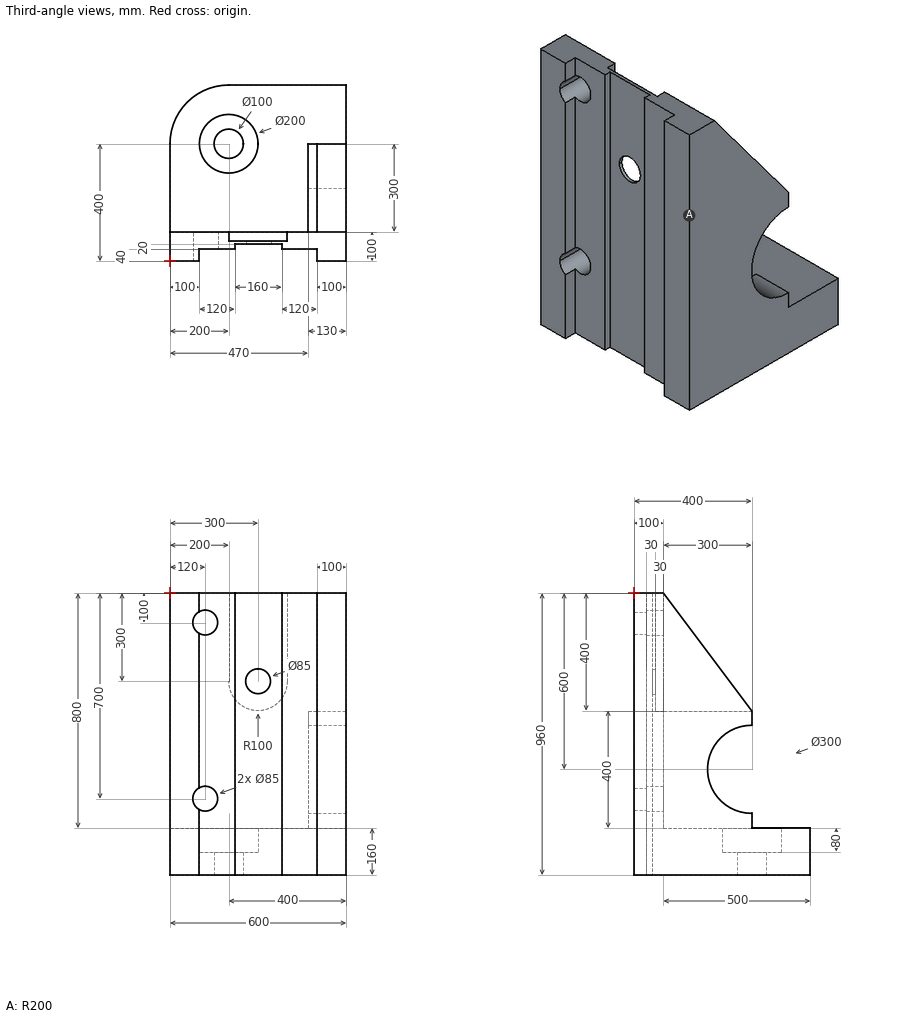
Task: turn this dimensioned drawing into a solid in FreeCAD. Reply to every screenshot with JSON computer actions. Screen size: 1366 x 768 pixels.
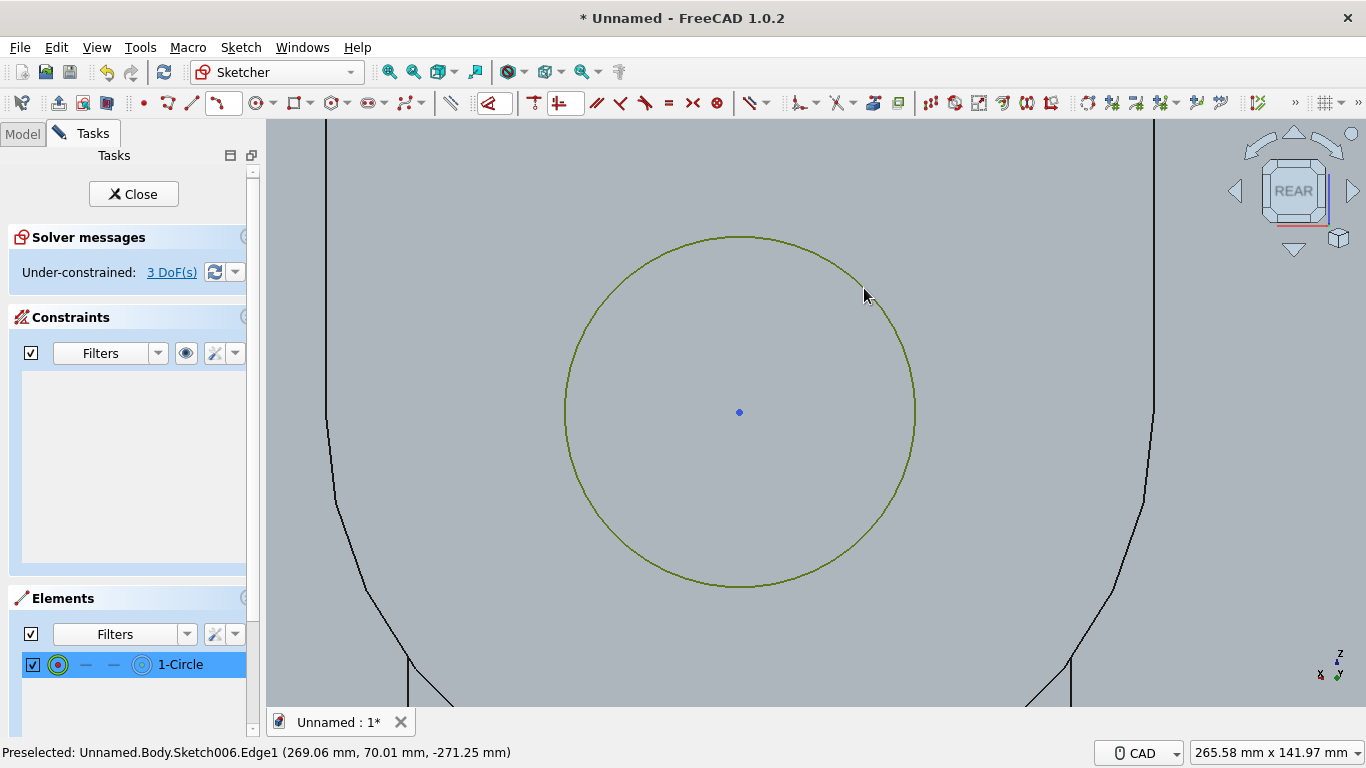
{"action": "key", "text": "k o"}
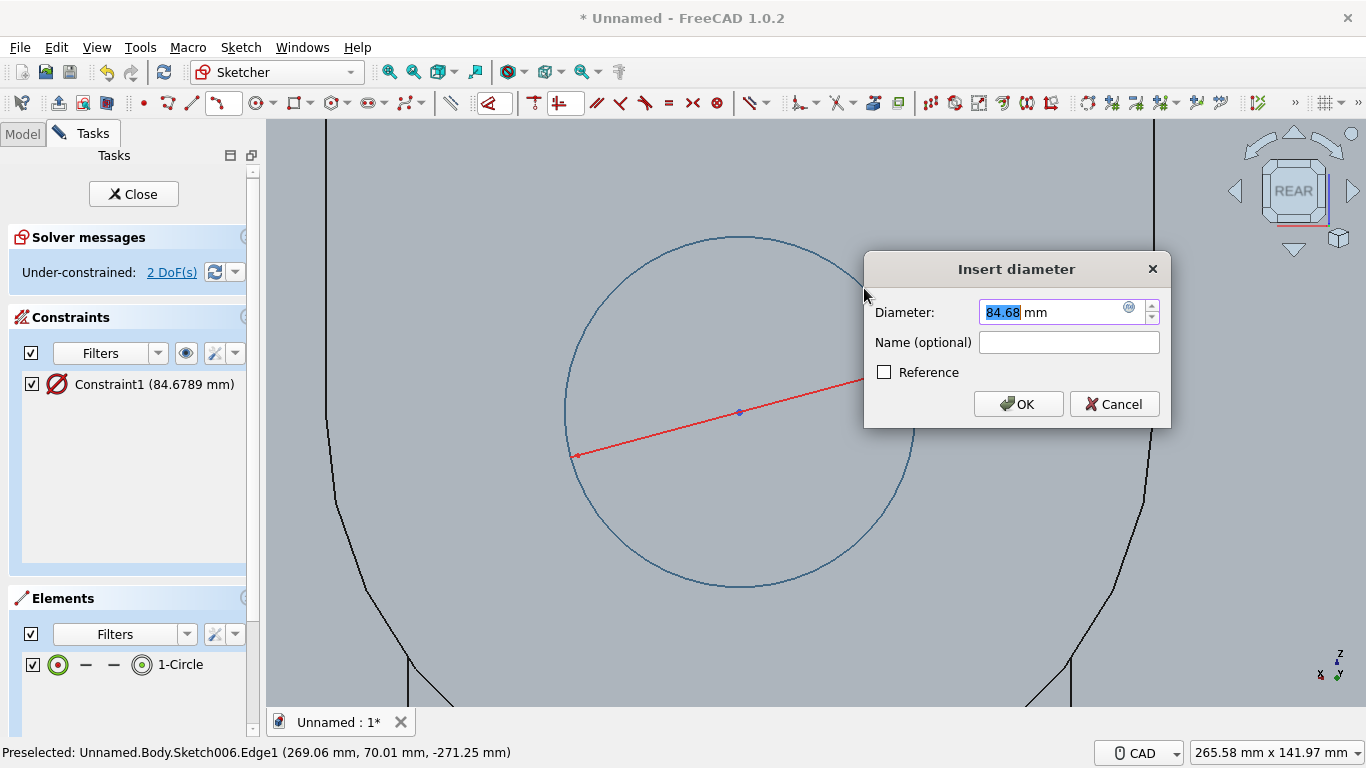
{"action": "type", "text": "85"}
{"action": "key", "text": "Return"}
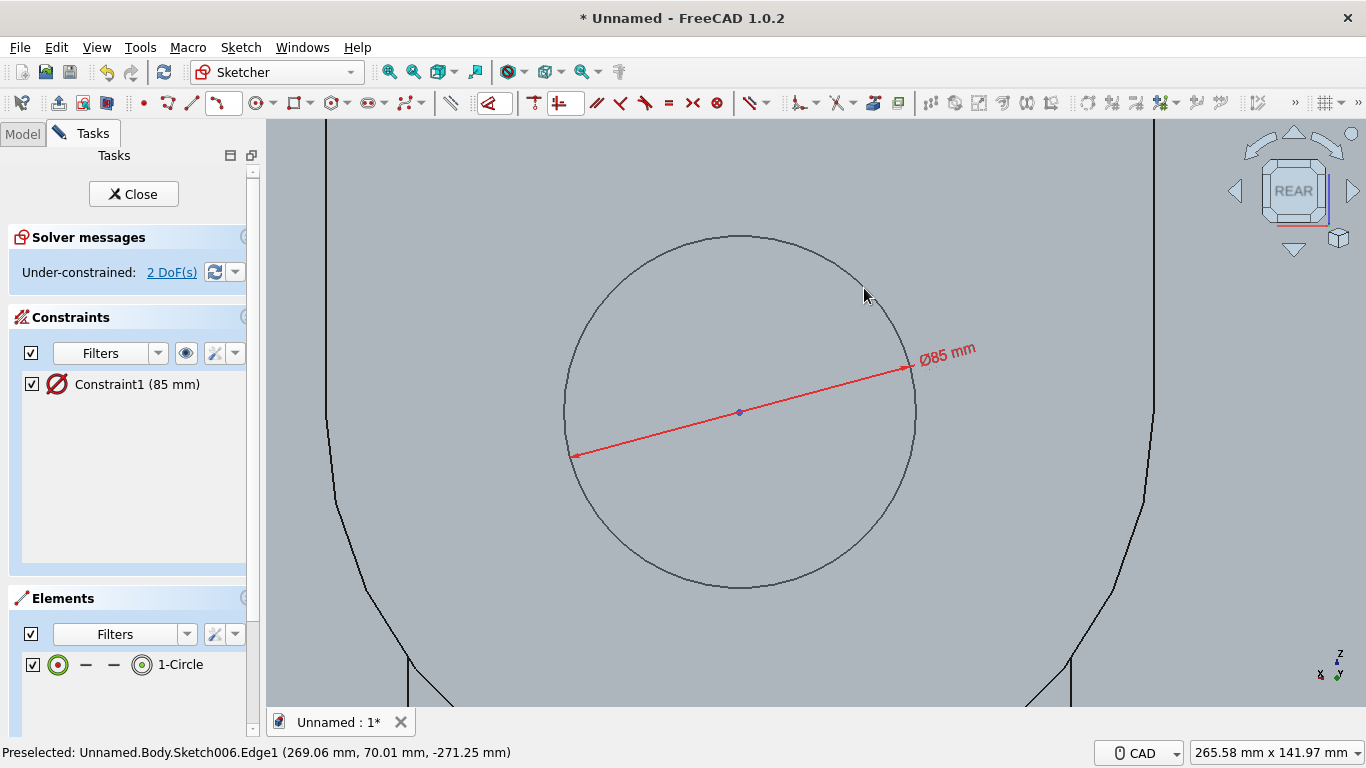
{"action": "left_click", "coordinate": [740, 412]}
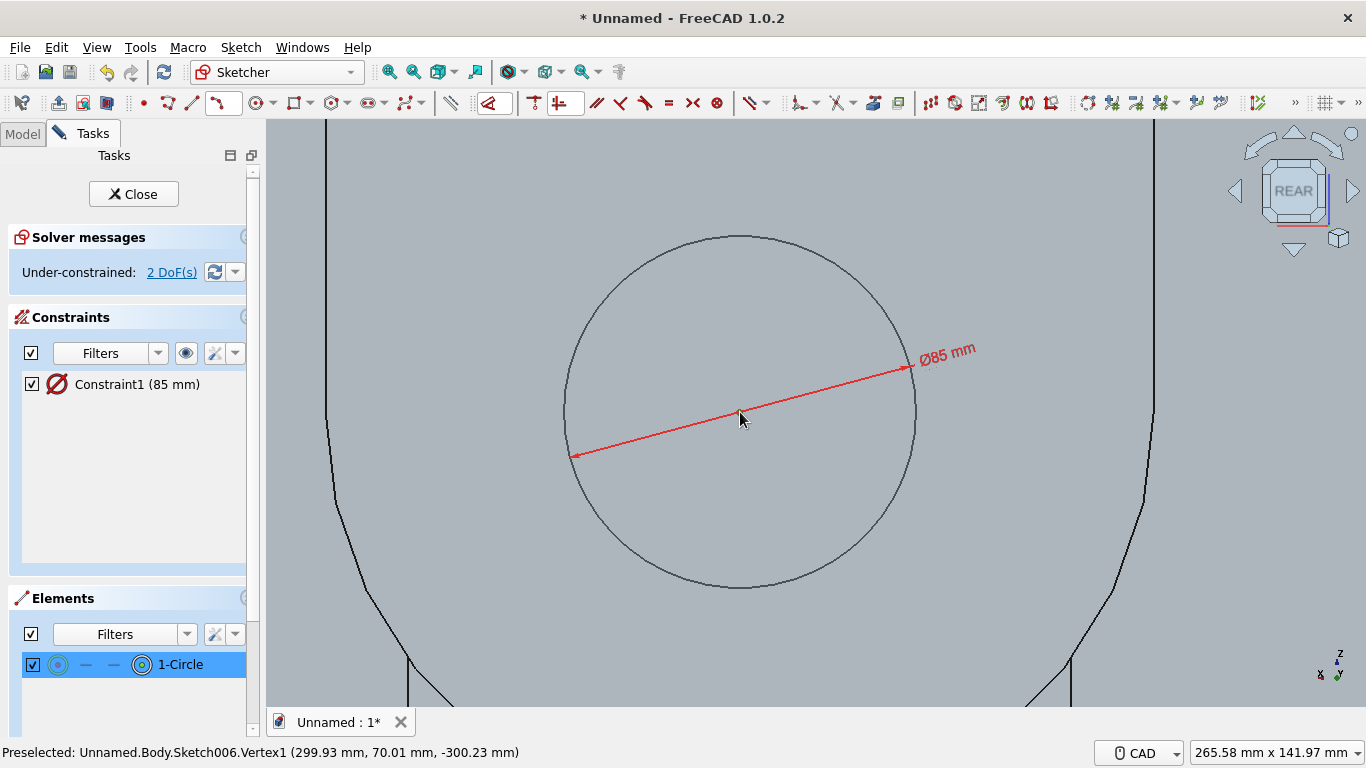
{"action": "left_click", "coordinate": [506, 104]}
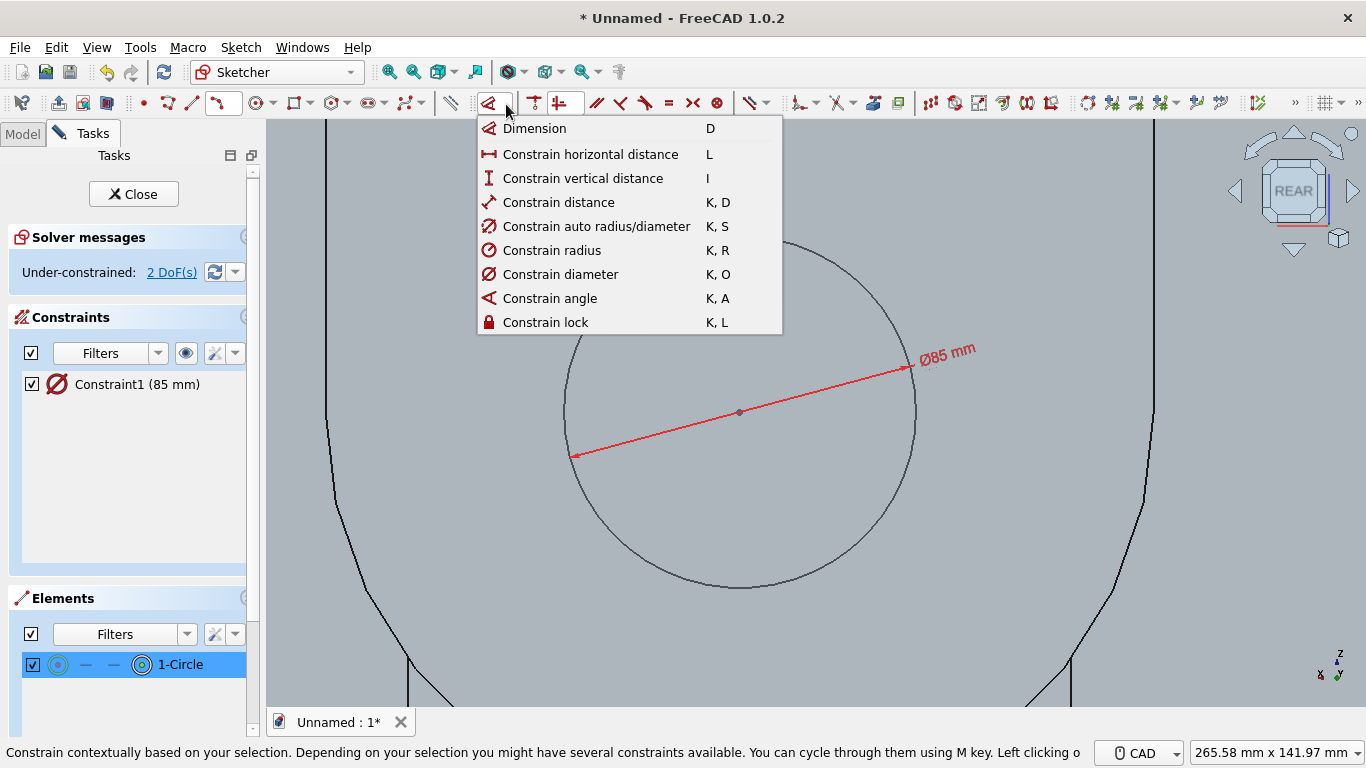
{"action": "left_click", "coordinate": [630, 154]}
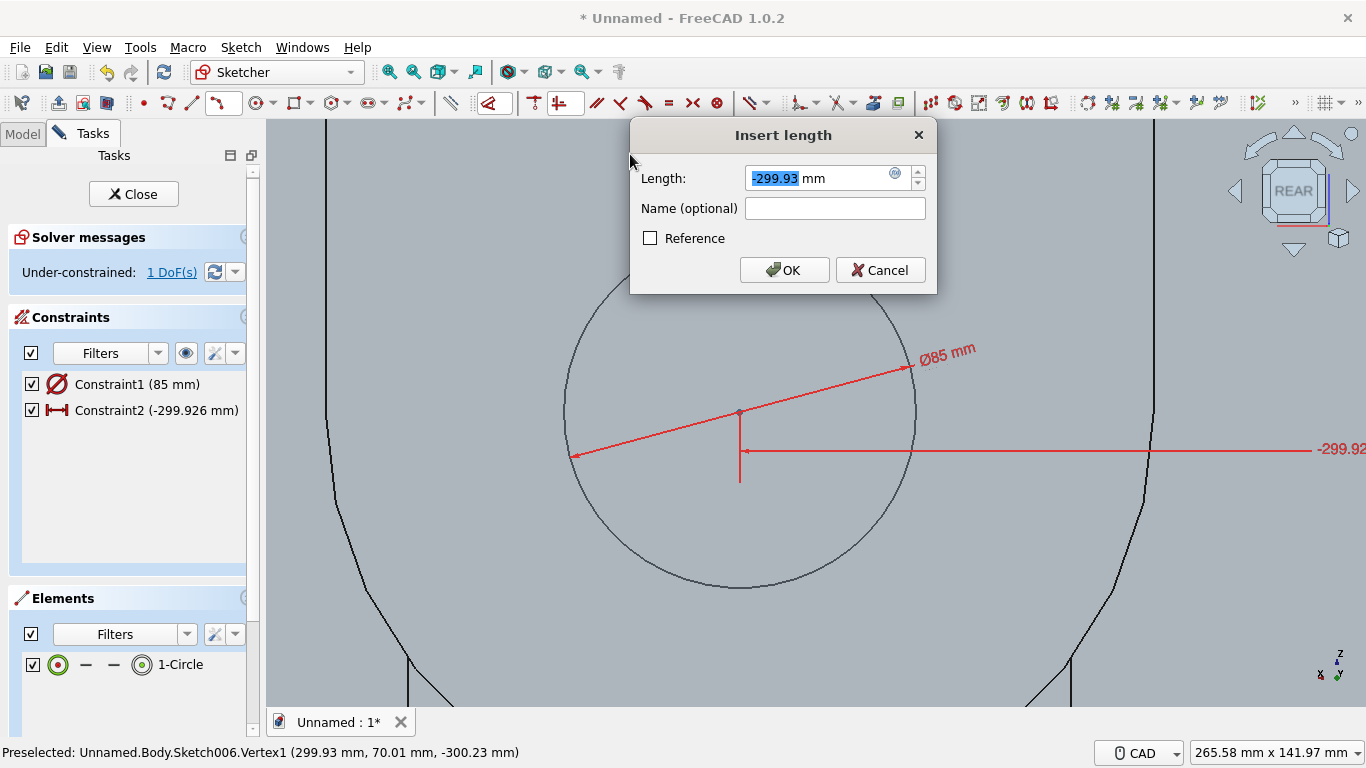
{"action": "type", "text": "-300"}
{"action": "key", "text": "Return"}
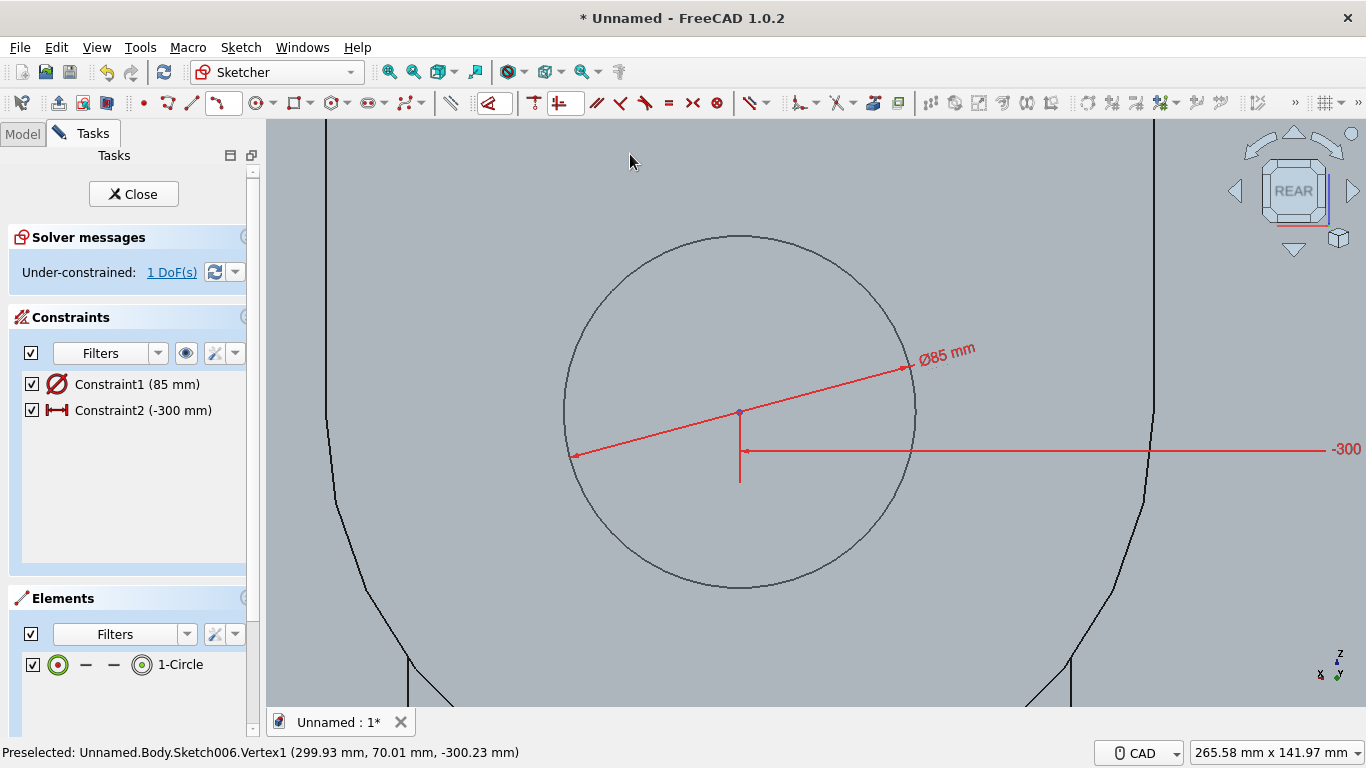
{"action": "left_click", "coordinate": [740, 412]}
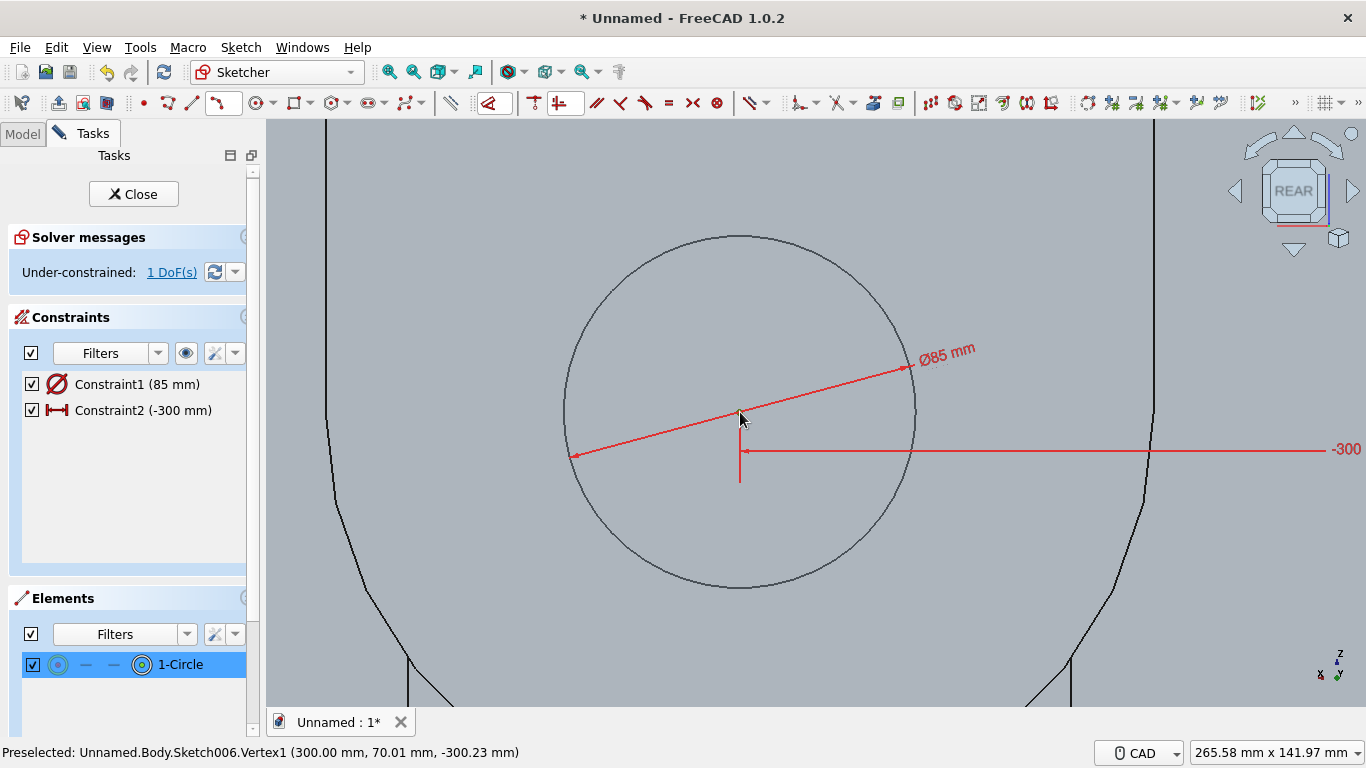
{"action": "left_click", "coordinate": [506, 104]}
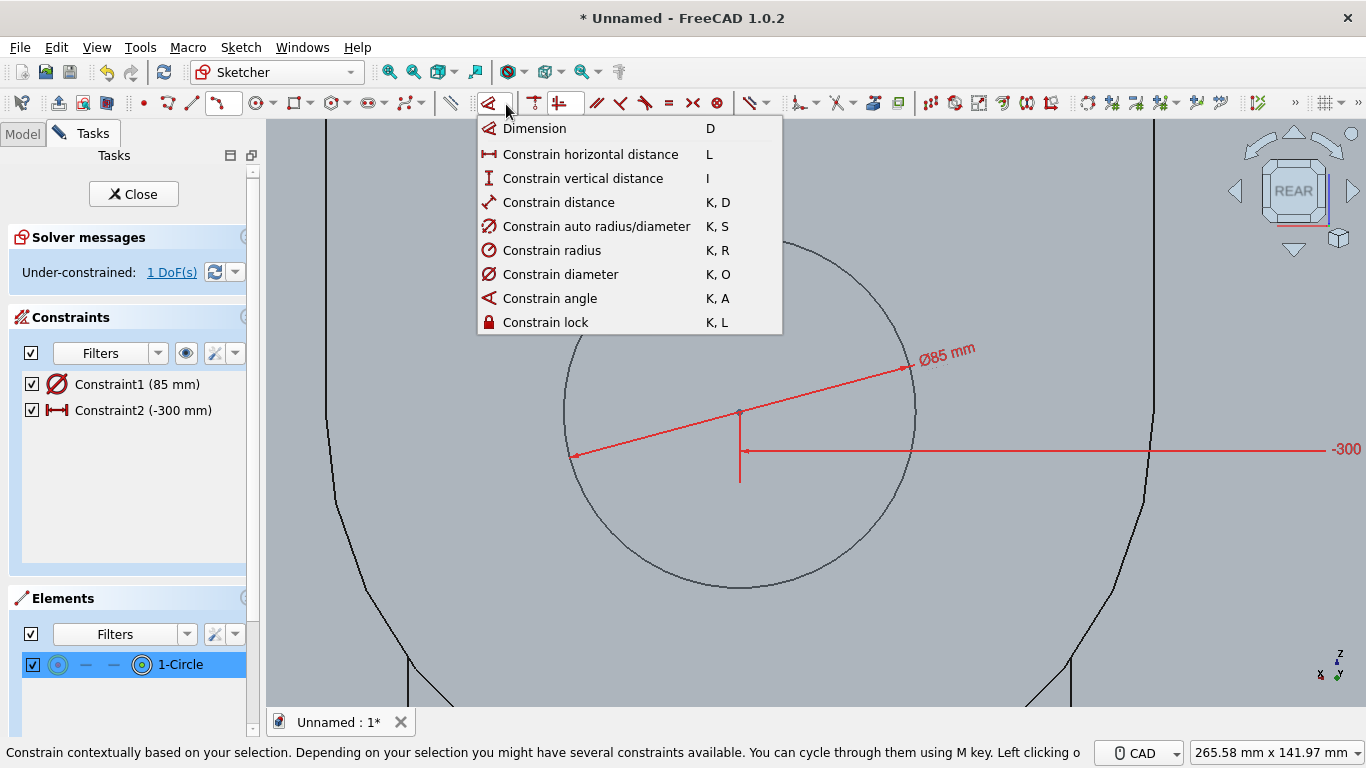
{"action": "left_click", "coordinate": [630, 178]}